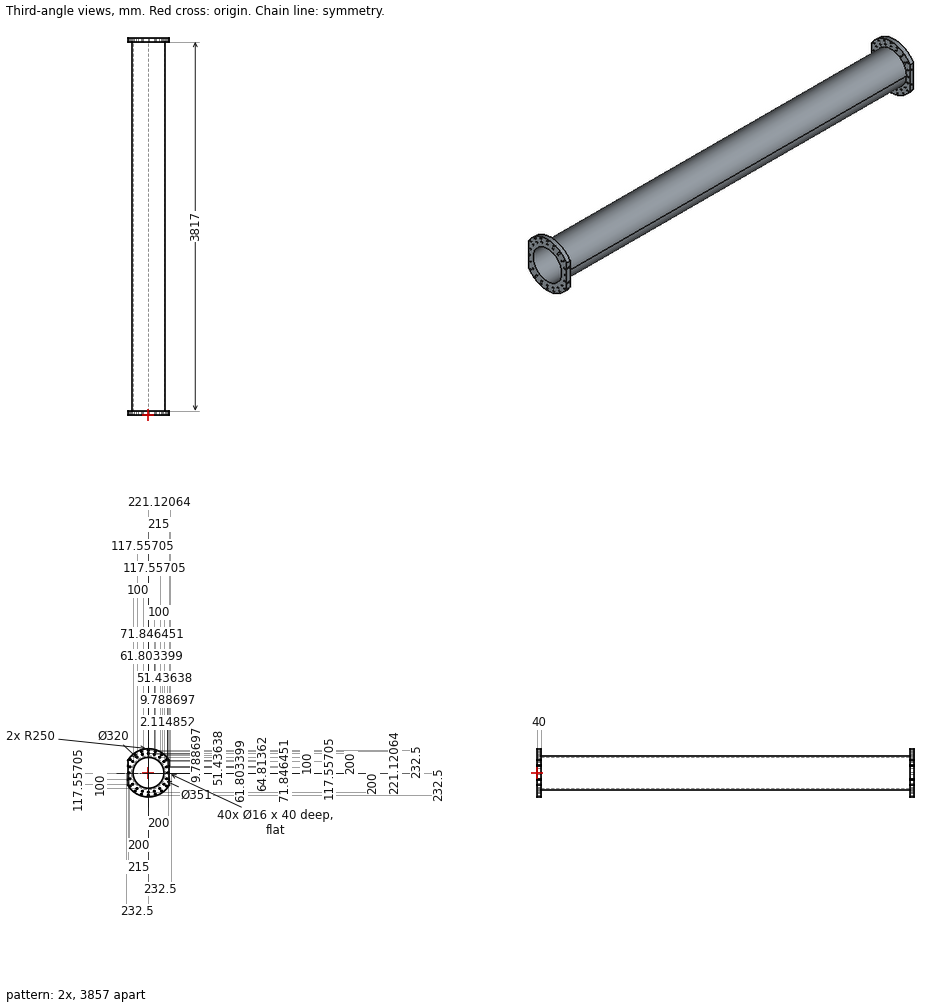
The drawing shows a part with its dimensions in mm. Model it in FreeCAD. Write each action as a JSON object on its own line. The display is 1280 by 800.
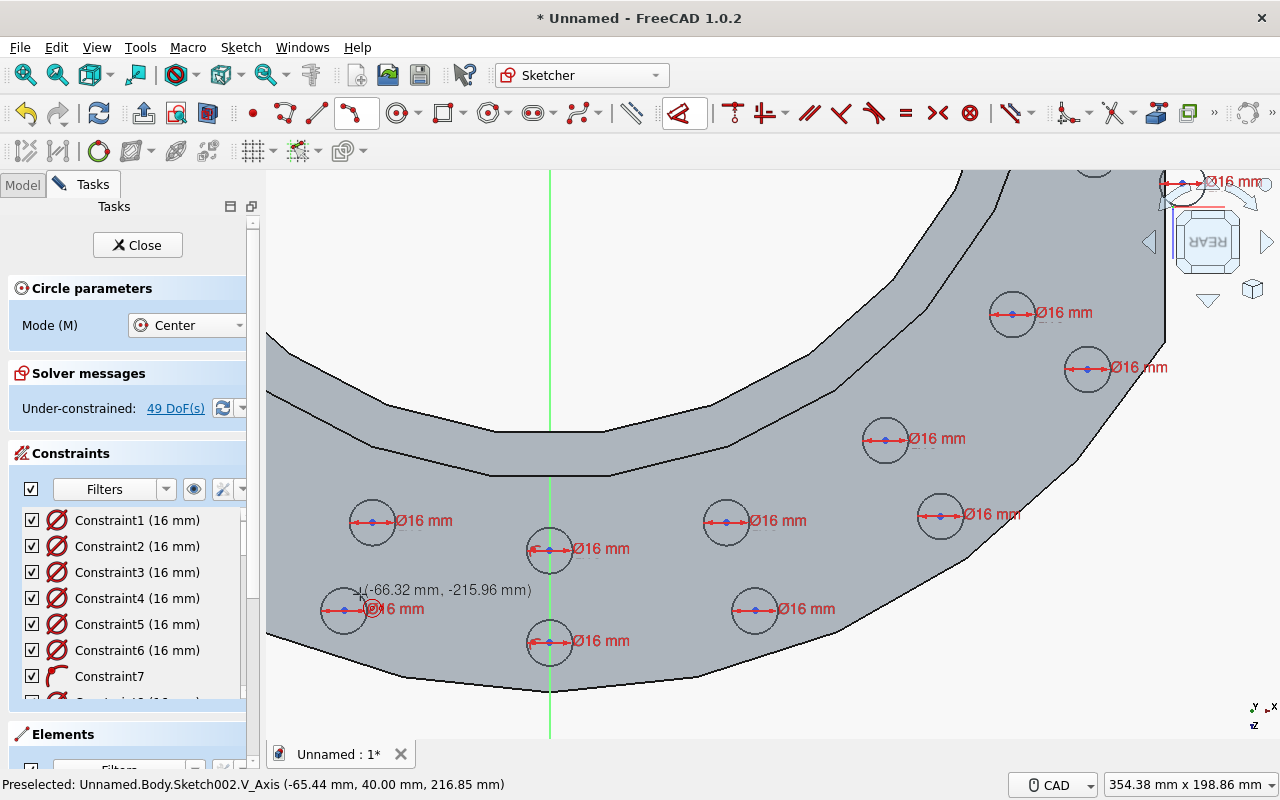
{"action": "scroll", "coordinate": [755, 611], "scroll_direction": "down", "scroll_amount": 7}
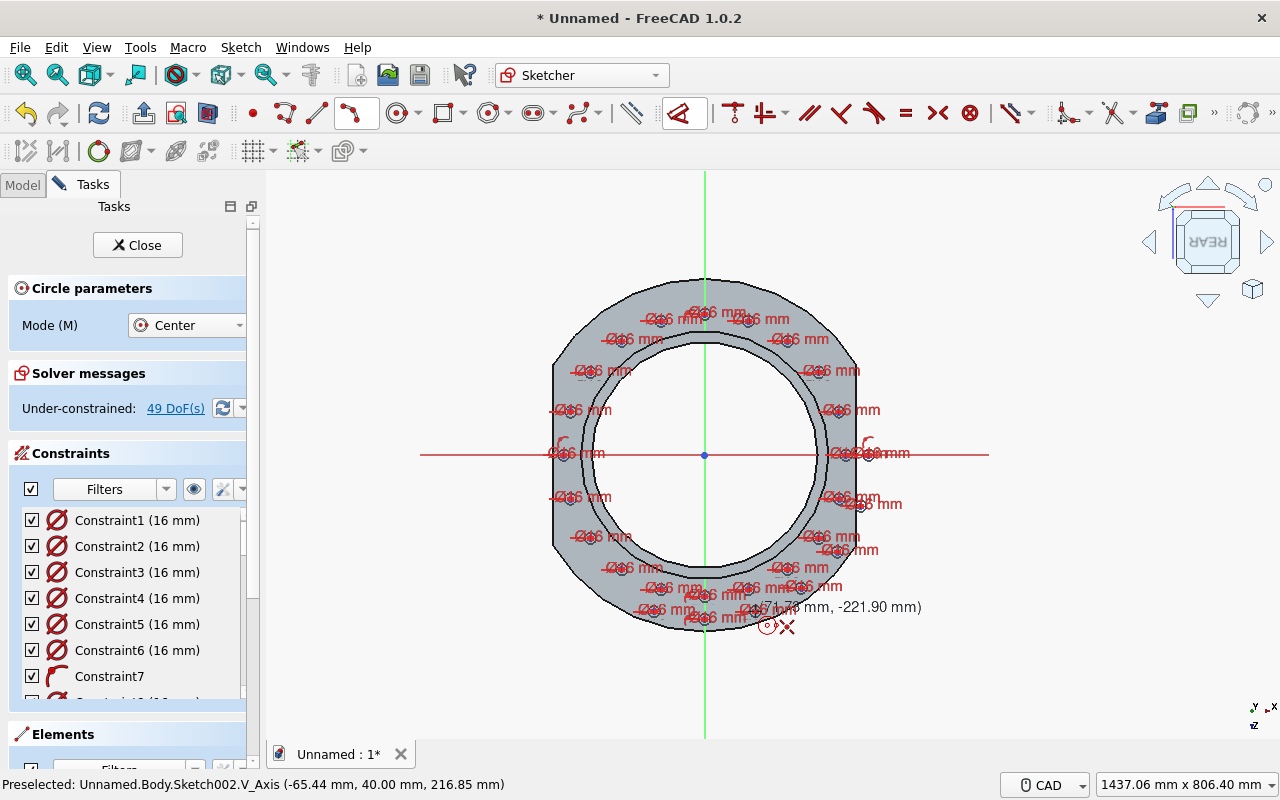
{"action": "scroll", "coordinate": [608, 588], "scroll_direction": "up", "scroll_amount": 7}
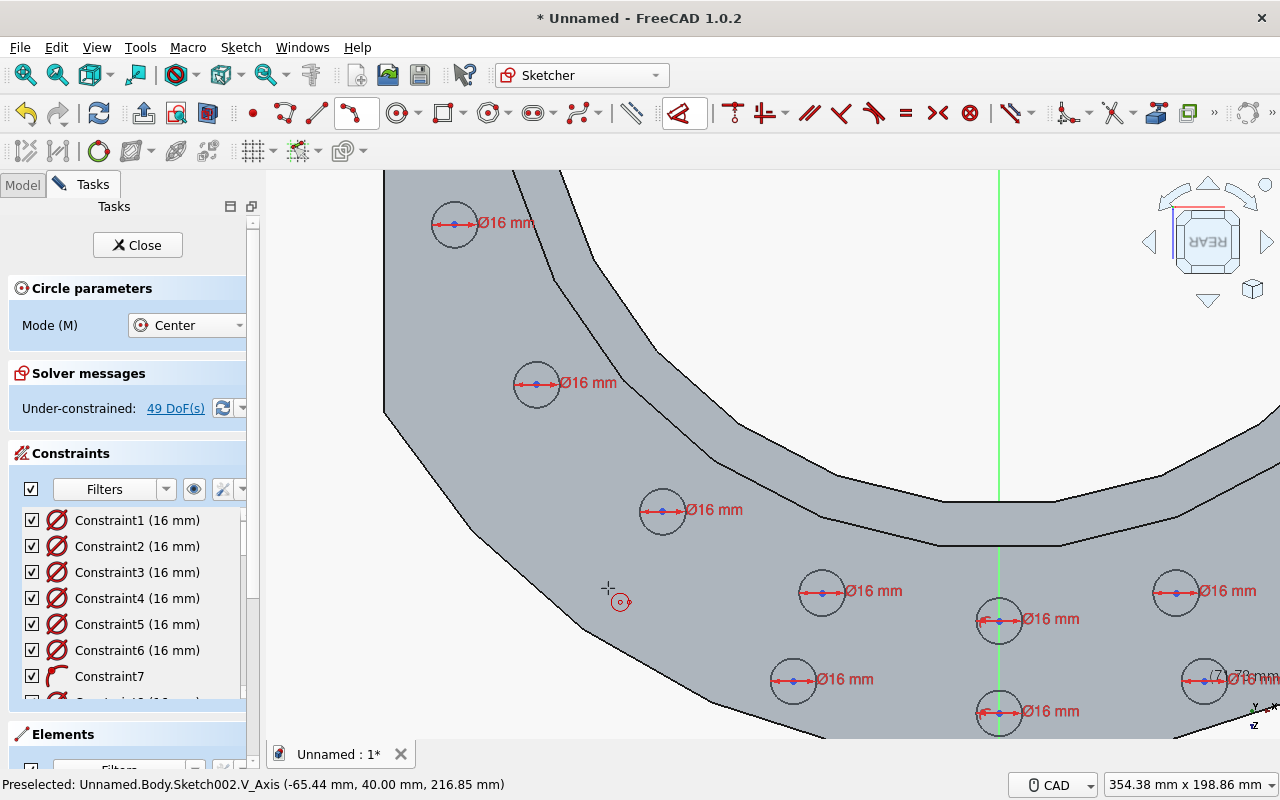
{"action": "left_click", "coordinate": [608, 586]}
{"action": "mouse_move", "coordinate": [624, 569]}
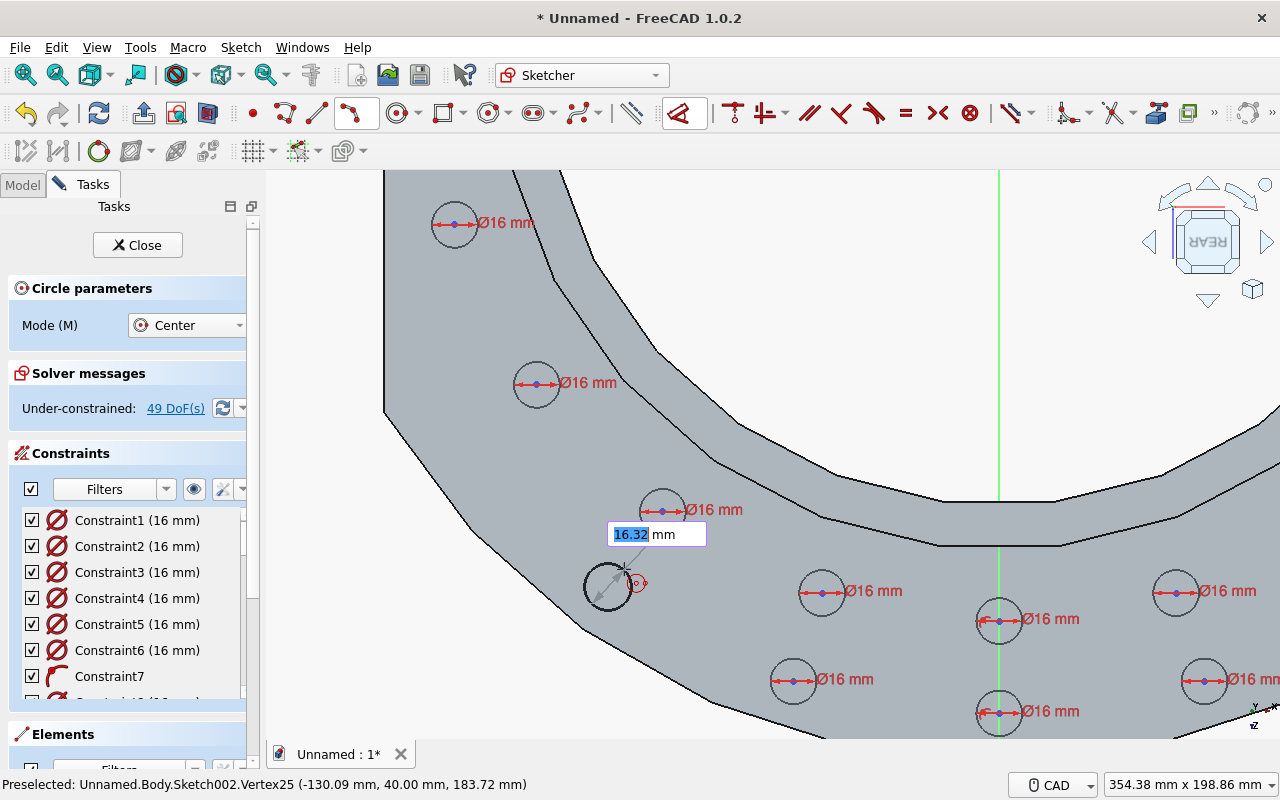
{"action": "type", "text": "16"}
{"action": "key", "text": "Return"}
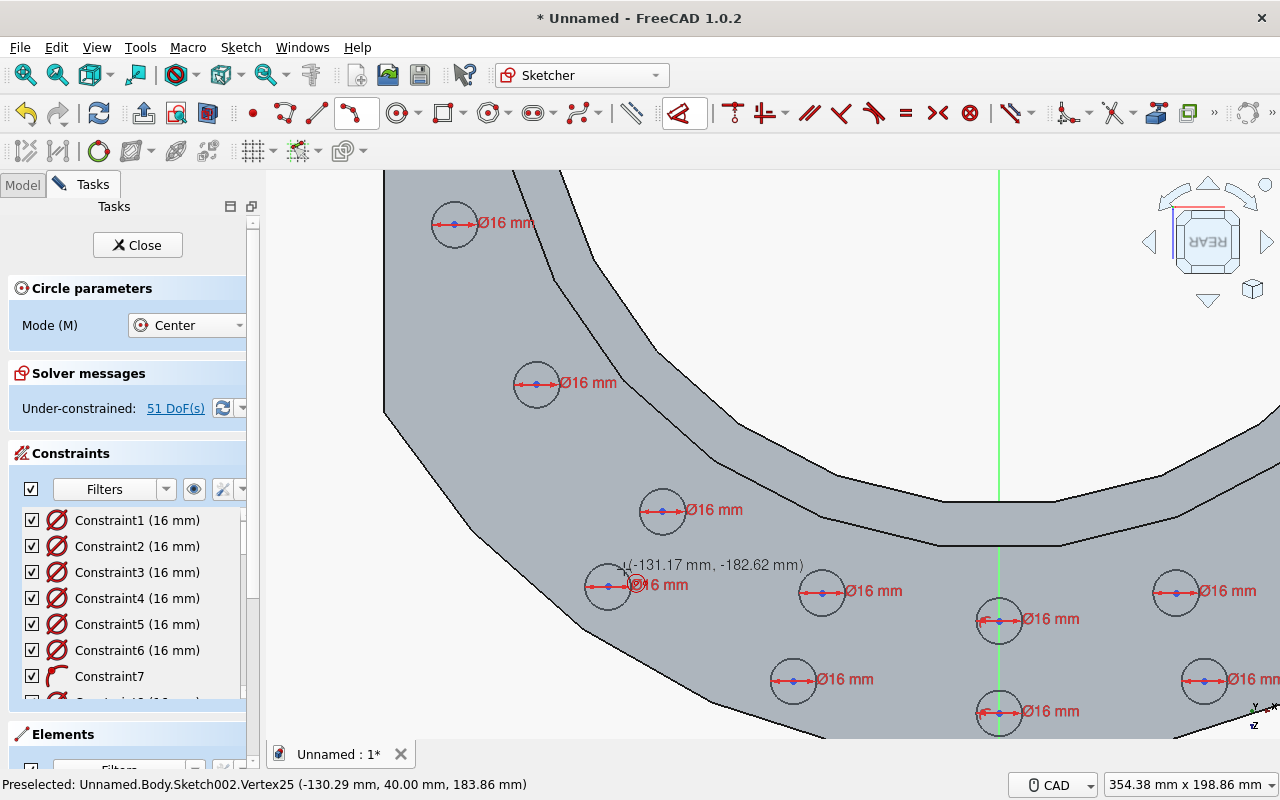
{"action": "left_click", "coordinate": [461, 438]}
{"action": "mouse_move", "coordinate": [477, 422]}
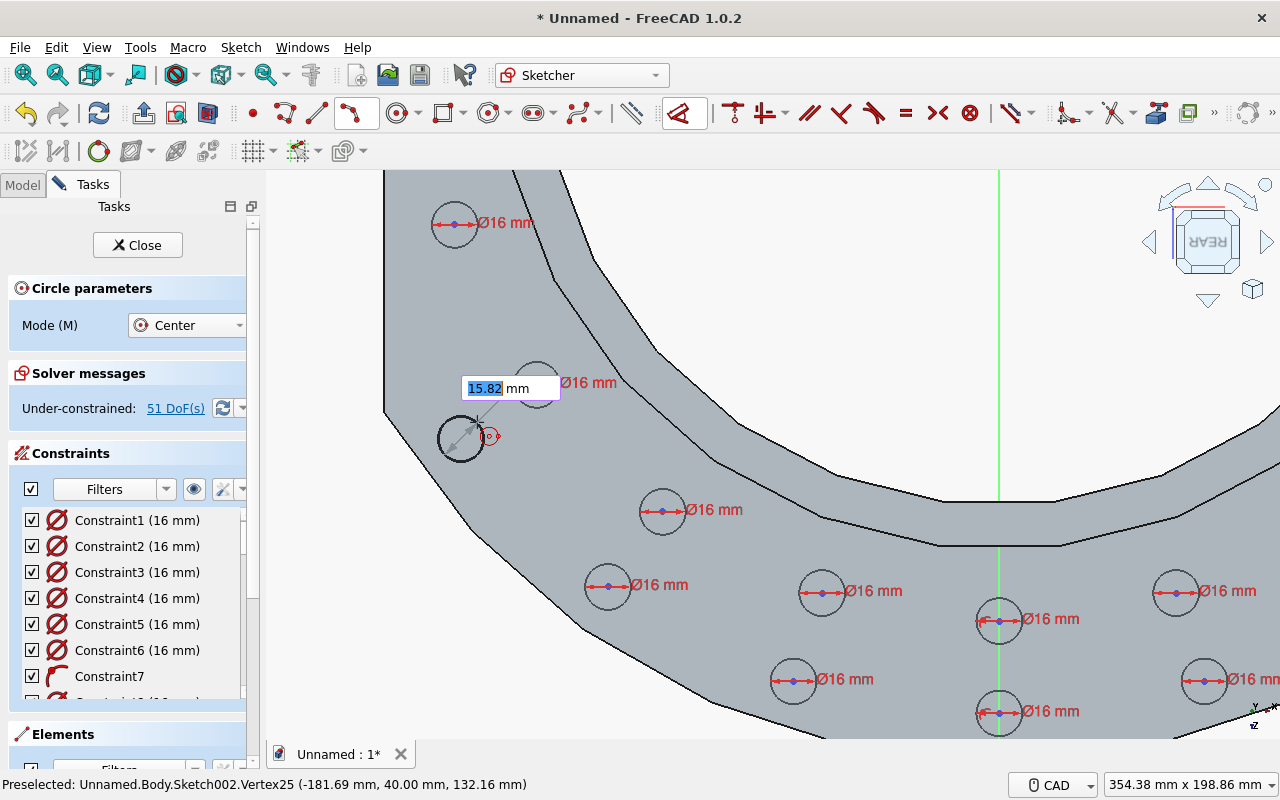
{"action": "type", "text": "16"}
{"action": "key", "text": "Return"}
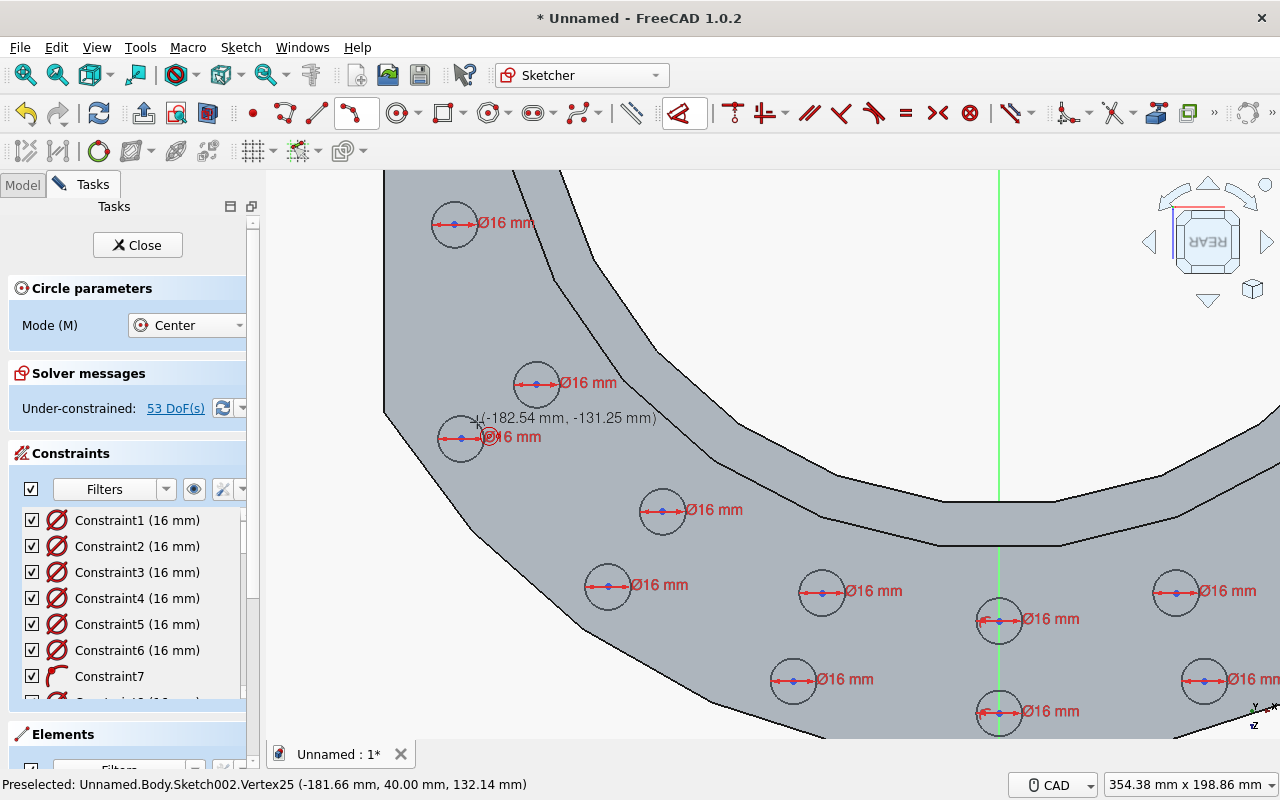
{"action": "left_click", "coordinate": [367, 253]}
{"action": "mouse_move", "coordinate": [383, 237]}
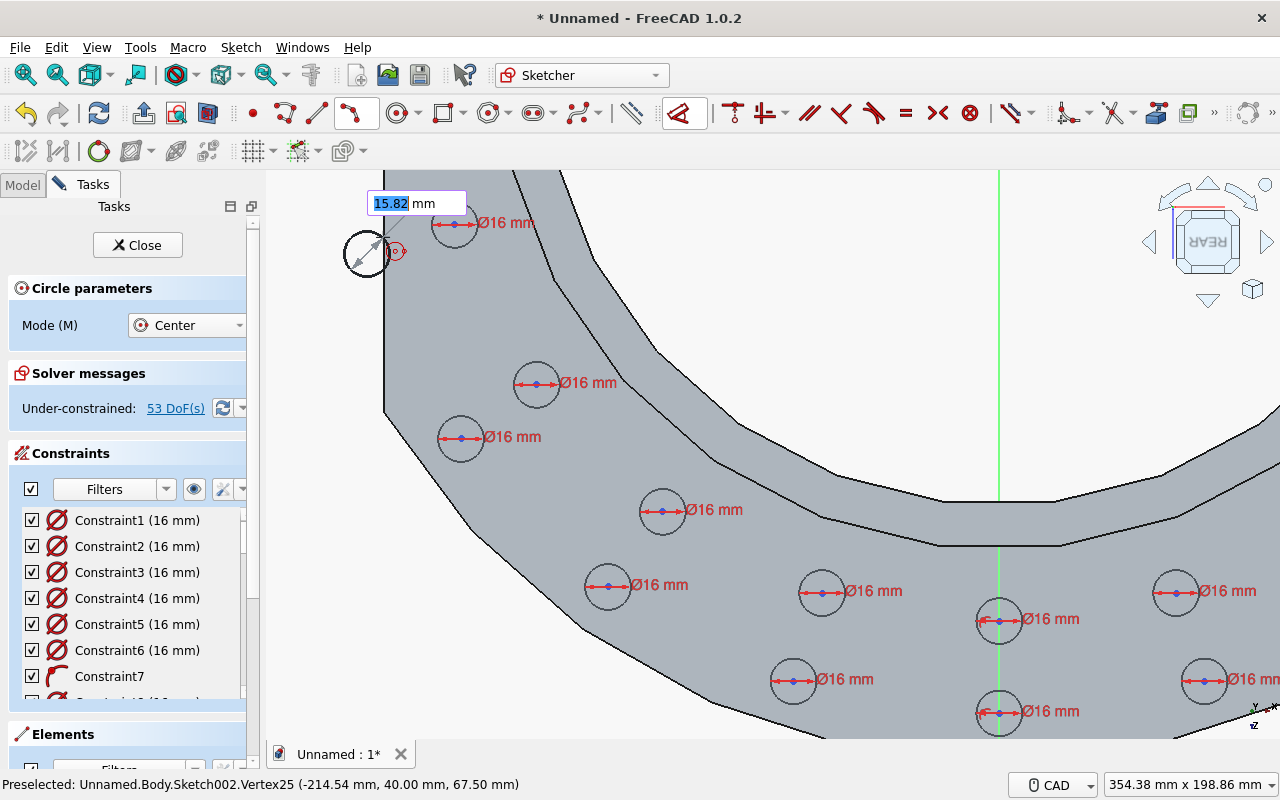
{"action": "type", "text": "16"}
{"action": "key", "text": "Return"}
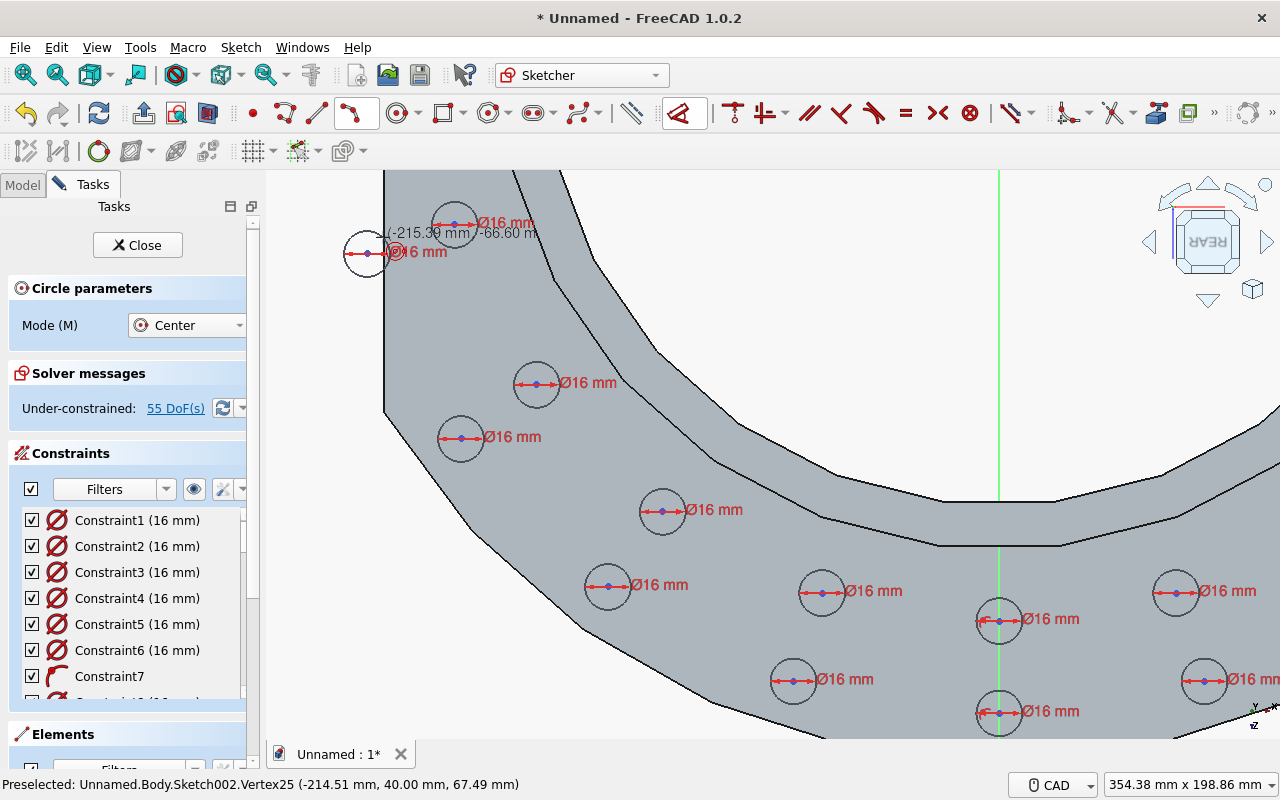
{"action": "scroll", "coordinate": [608, 588], "scroll_direction": "down", "scroll_amount": 7}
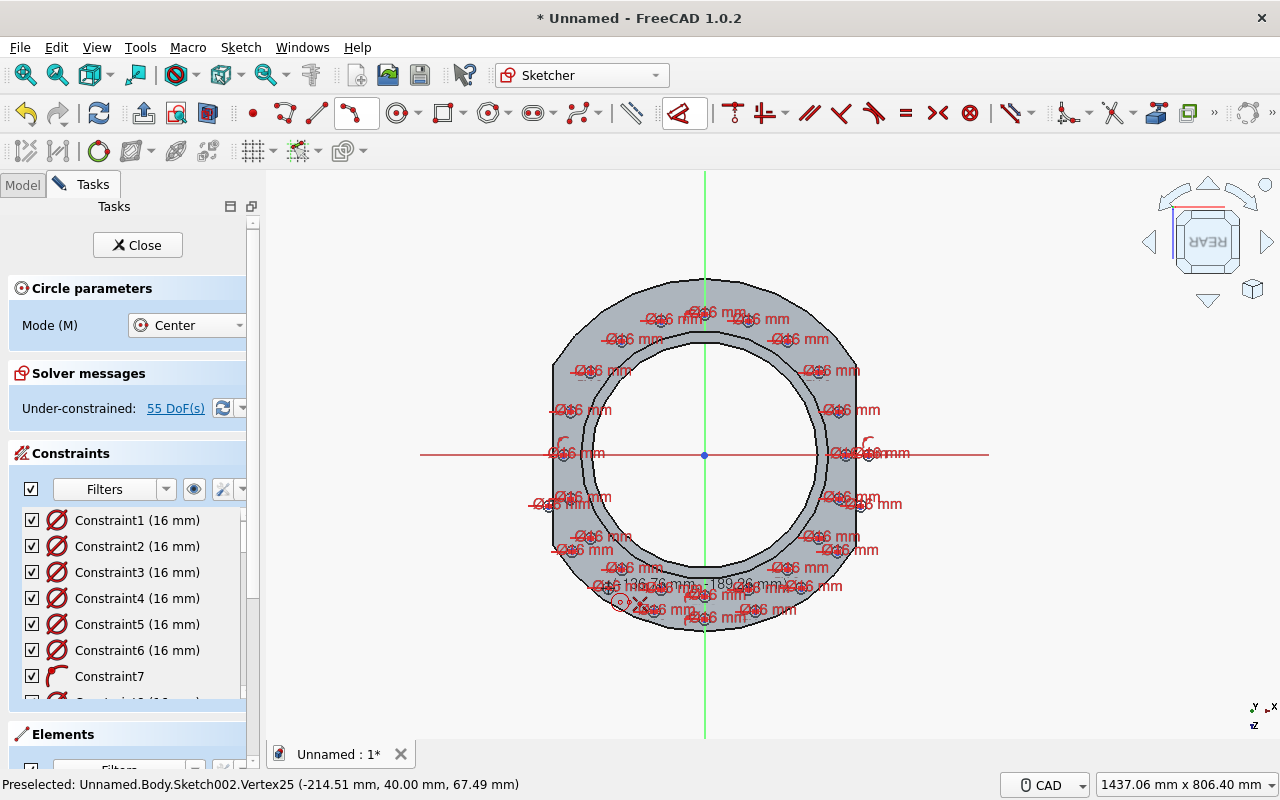
{"action": "scroll", "coordinate": [541, 455], "scroll_direction": "up", "scroll_amount": 7}